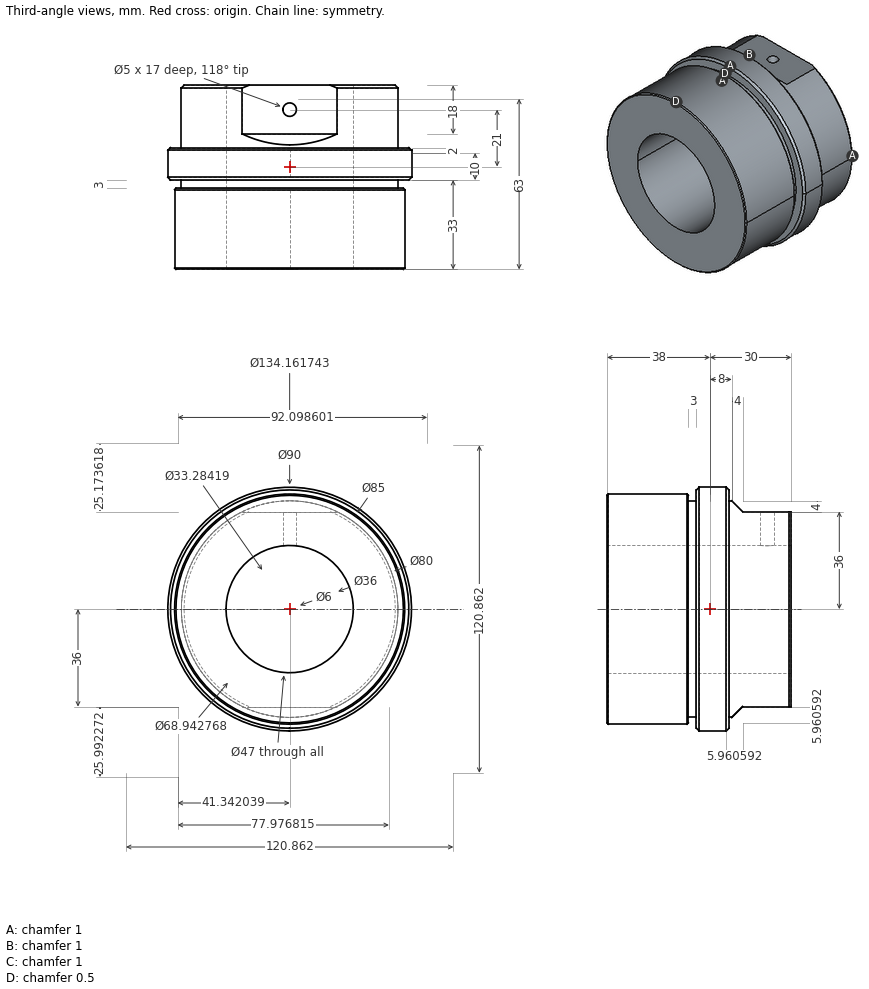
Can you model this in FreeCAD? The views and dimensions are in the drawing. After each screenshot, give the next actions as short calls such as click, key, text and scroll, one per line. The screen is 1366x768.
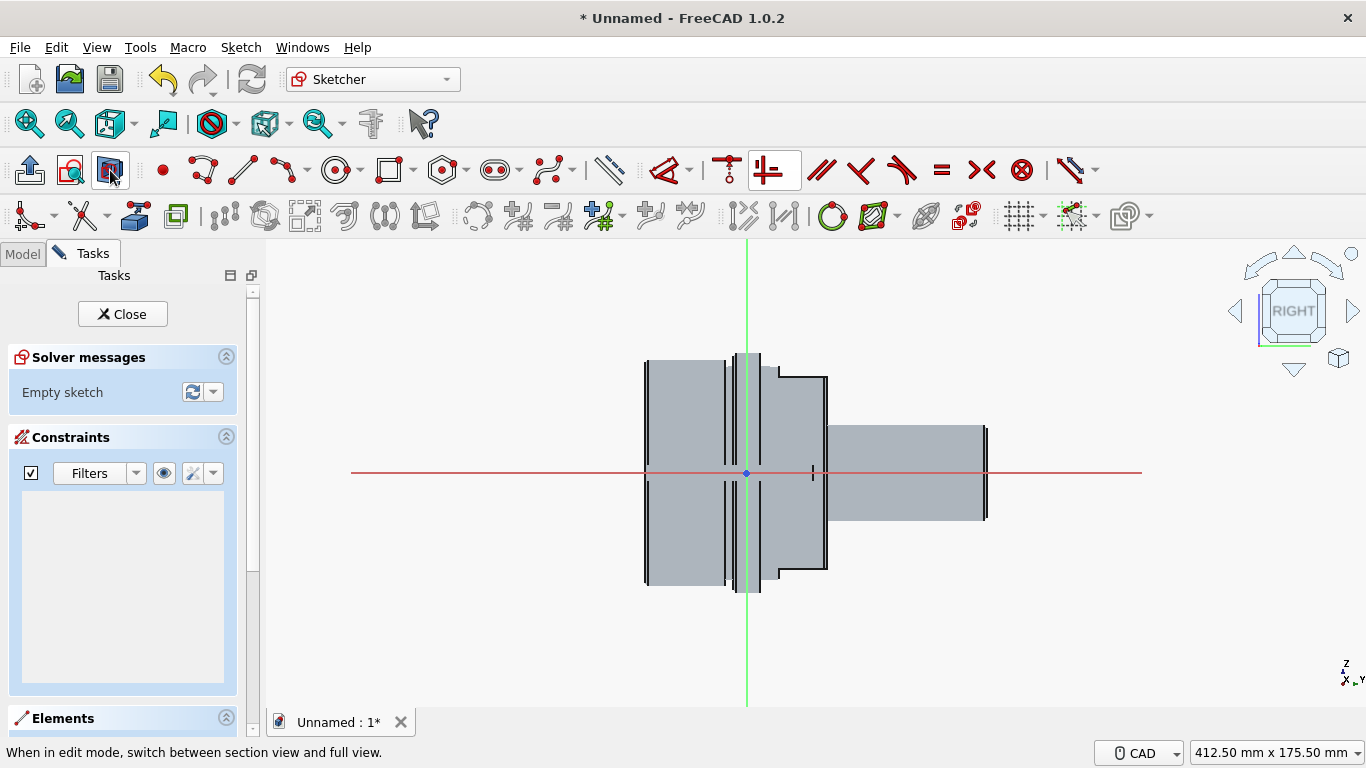
click(204, 170)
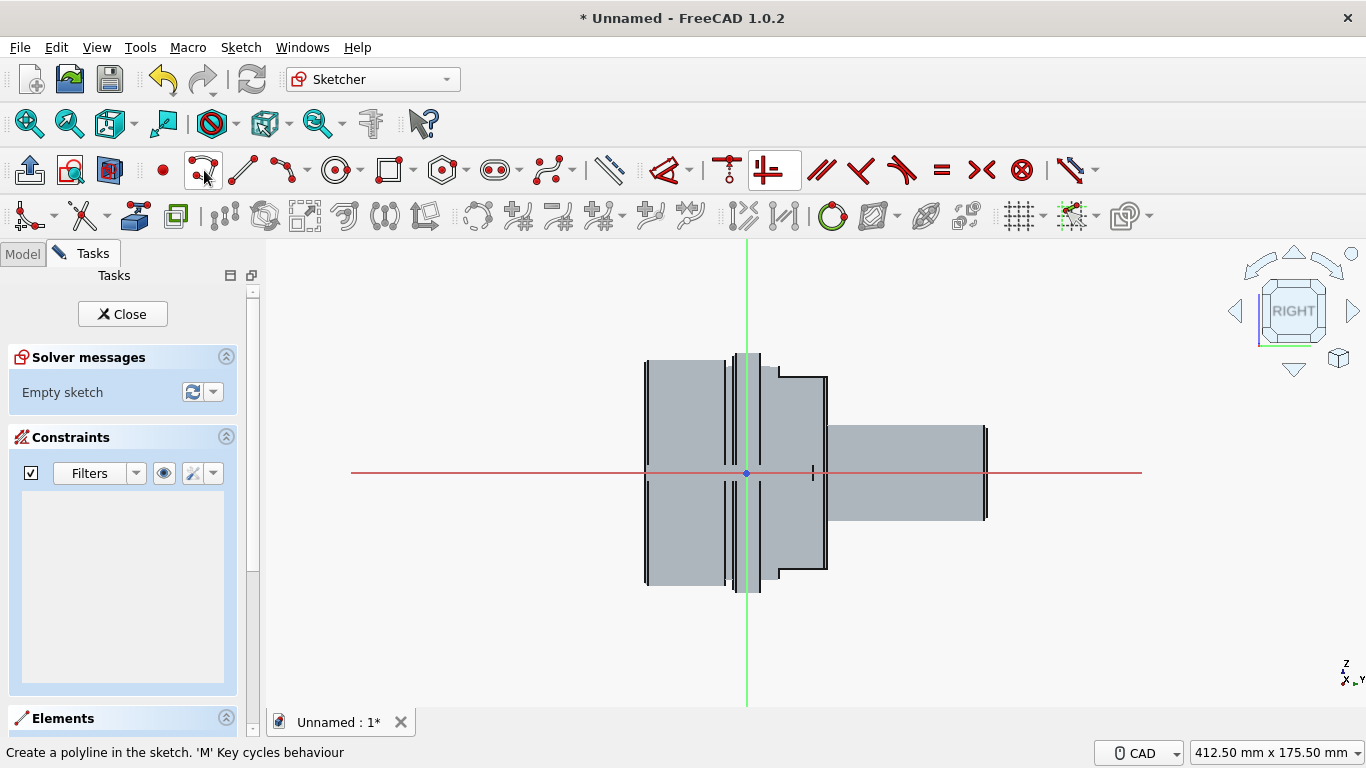
click(779, 377)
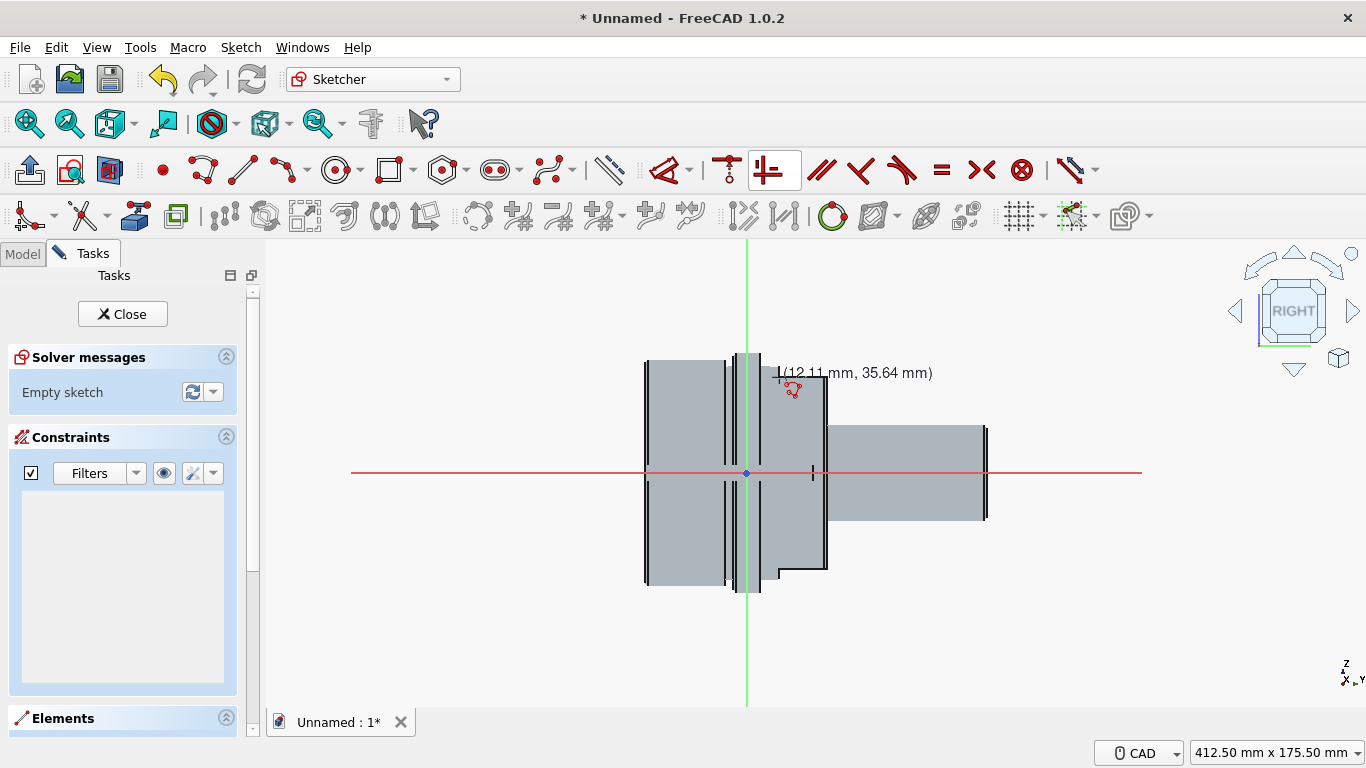
scroll(779, 366, up, 2)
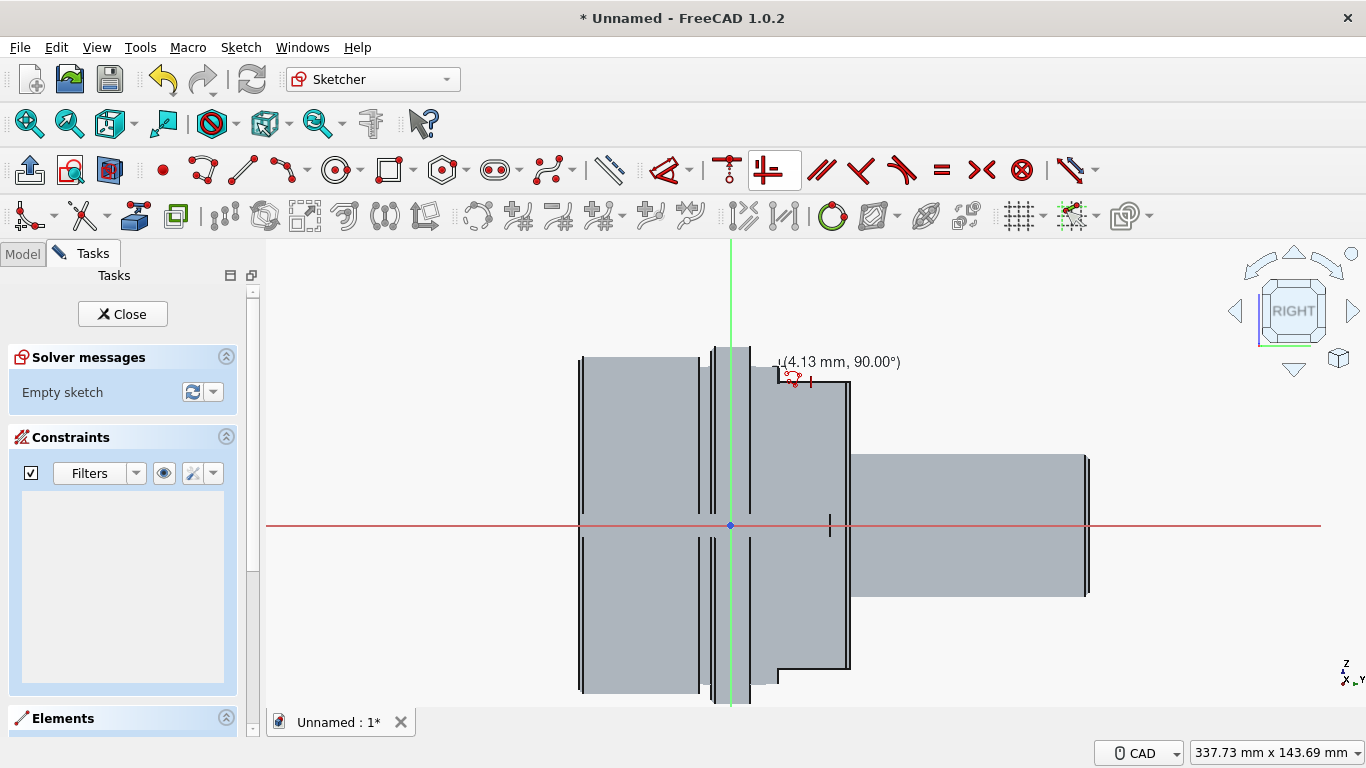
click(779, 366)
click(762, 366)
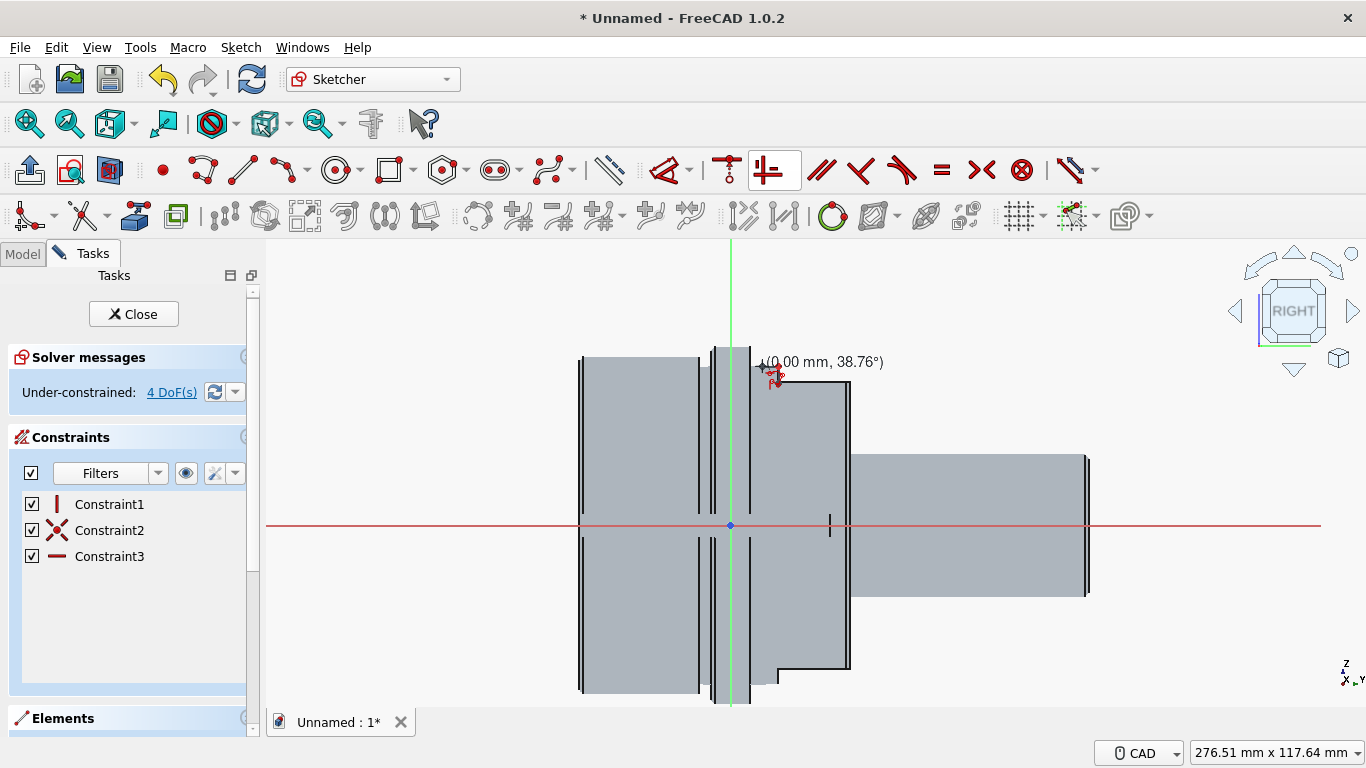
scroll(778, 382, up, 4)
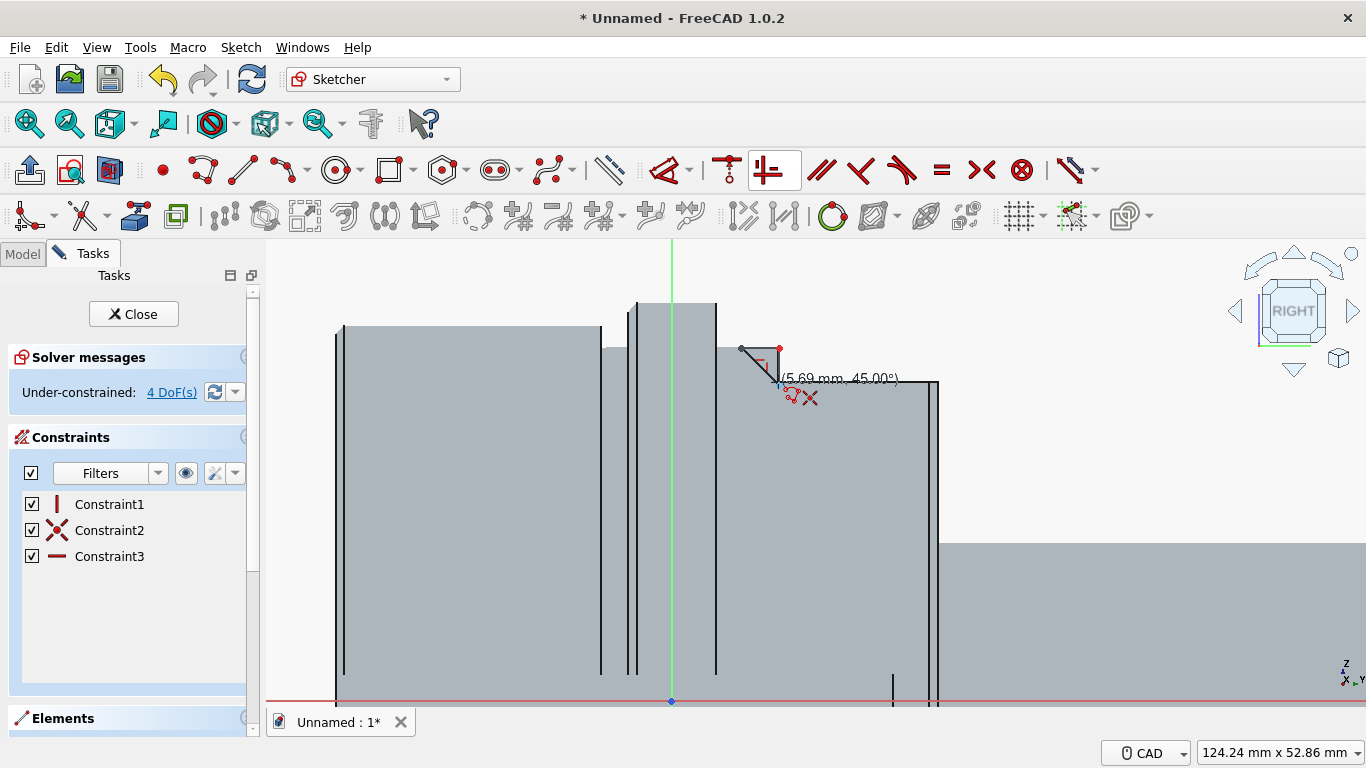
click(779, 386)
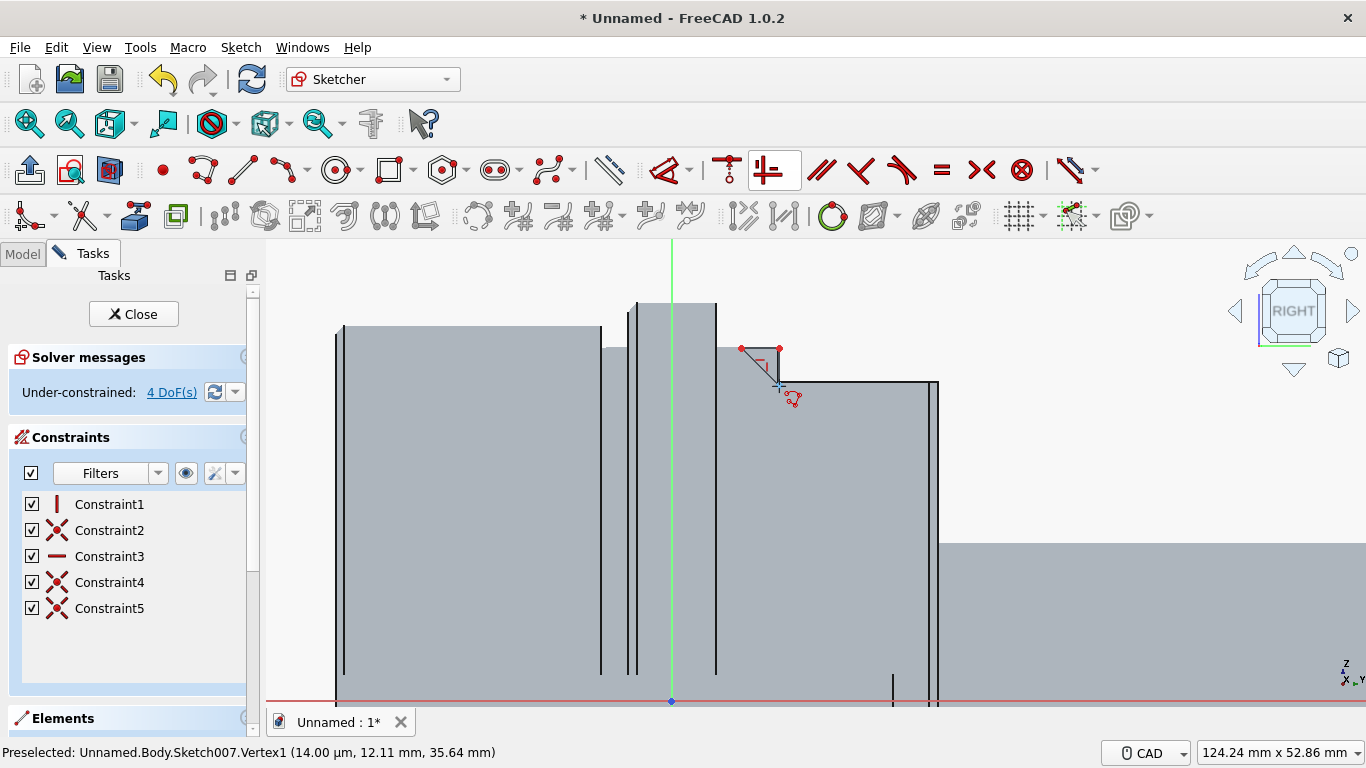
scroll(761, 335, down, 5)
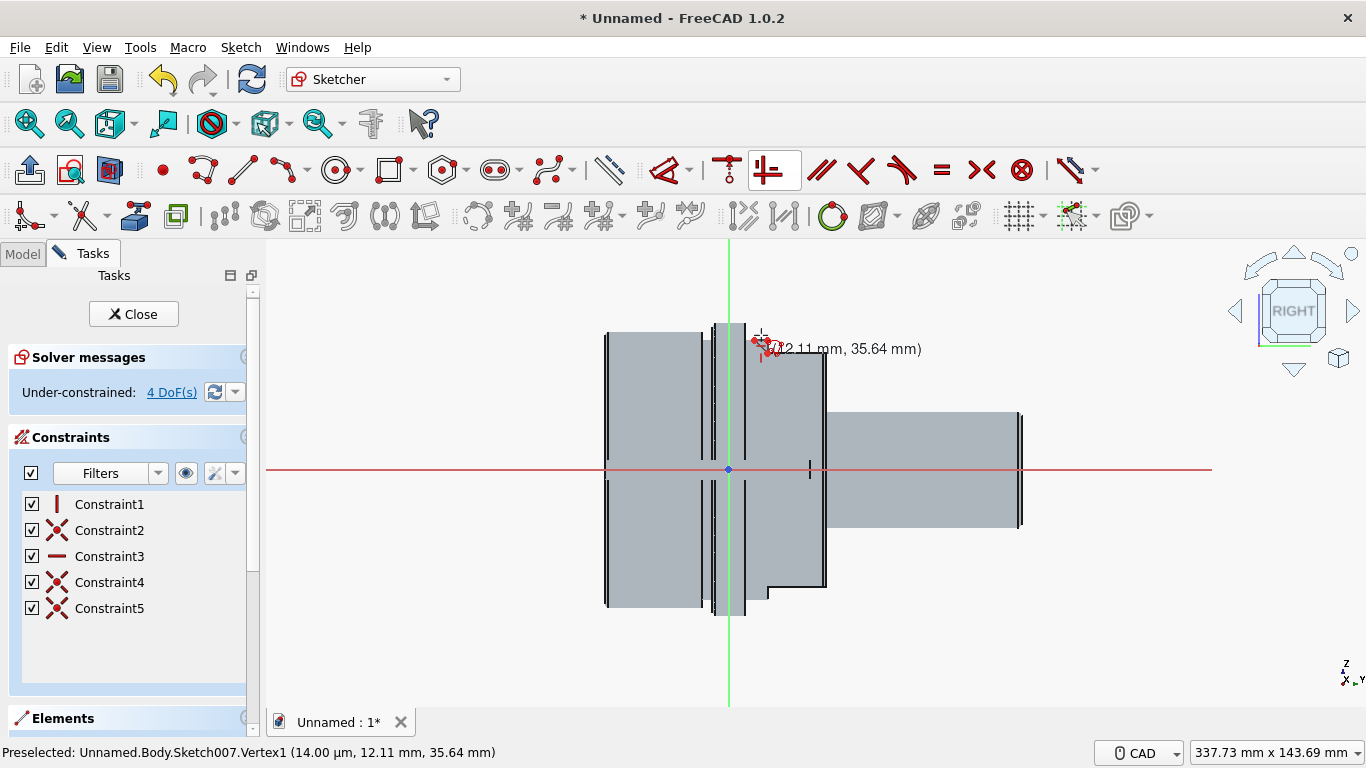
click(768, 587)
click(748, 606)
click(768, 606)
click(768, 588)
key(Escape)
key(Escape)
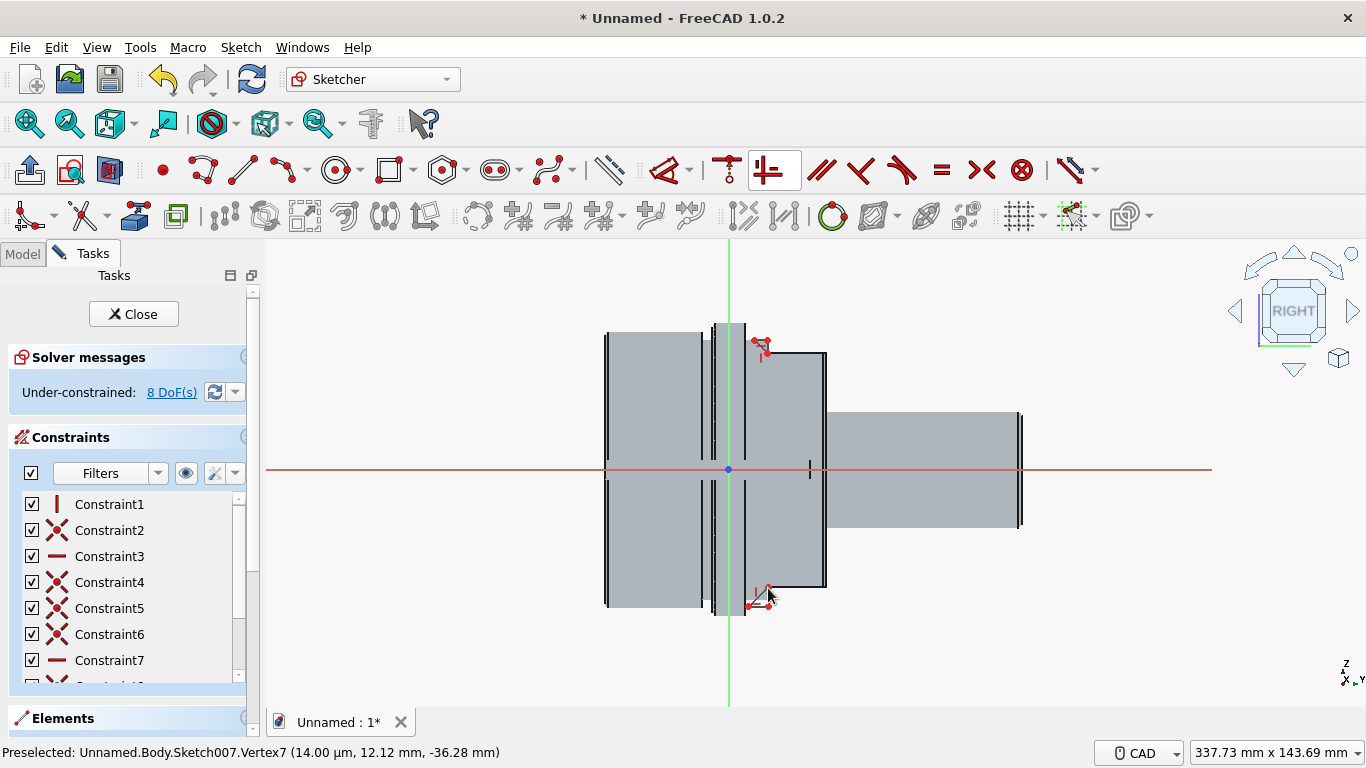
click(768, 354)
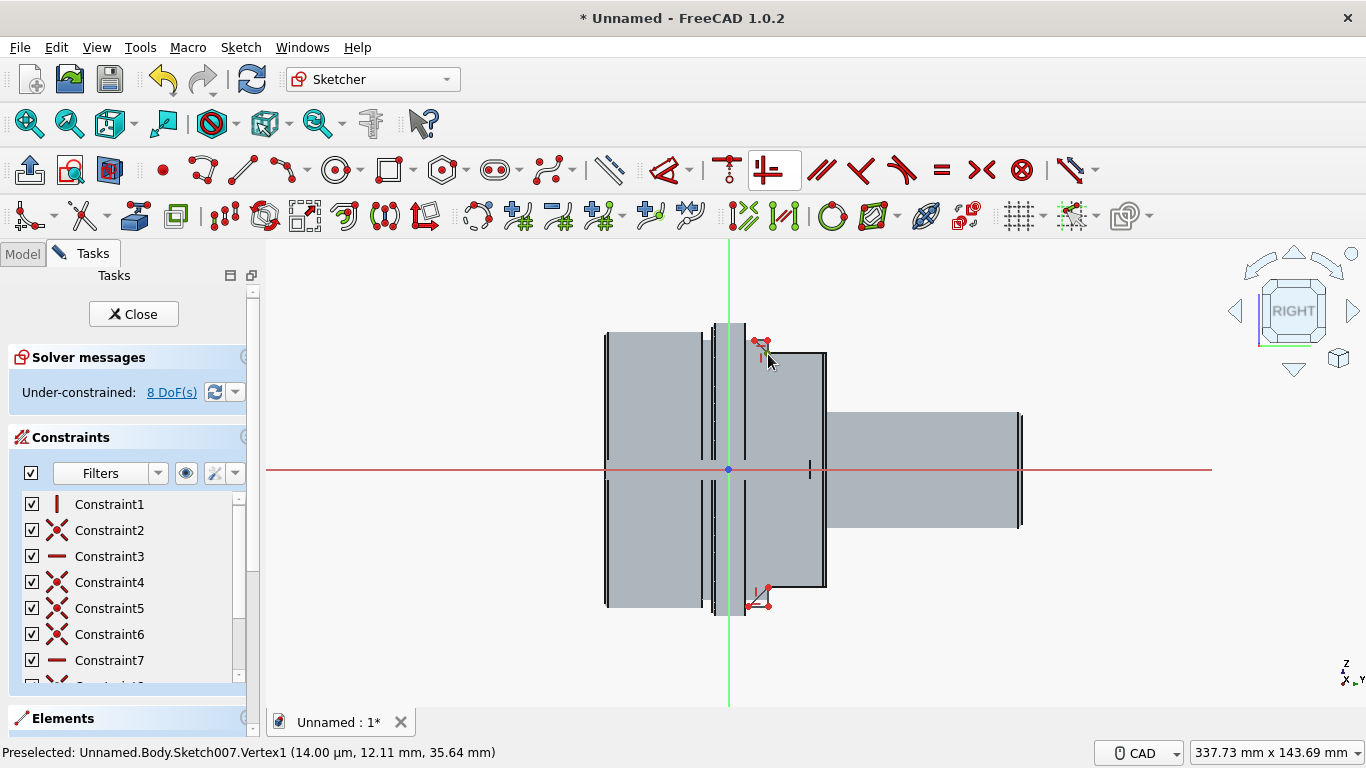
click(768, 588)